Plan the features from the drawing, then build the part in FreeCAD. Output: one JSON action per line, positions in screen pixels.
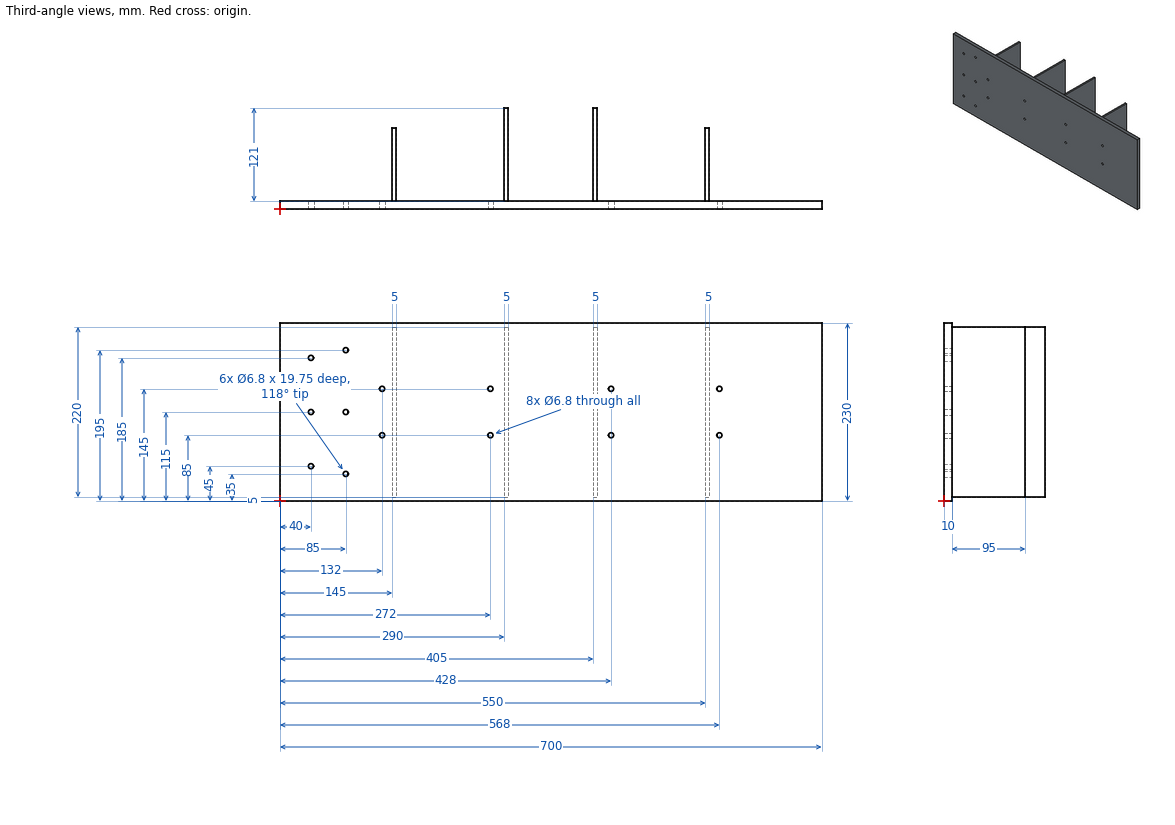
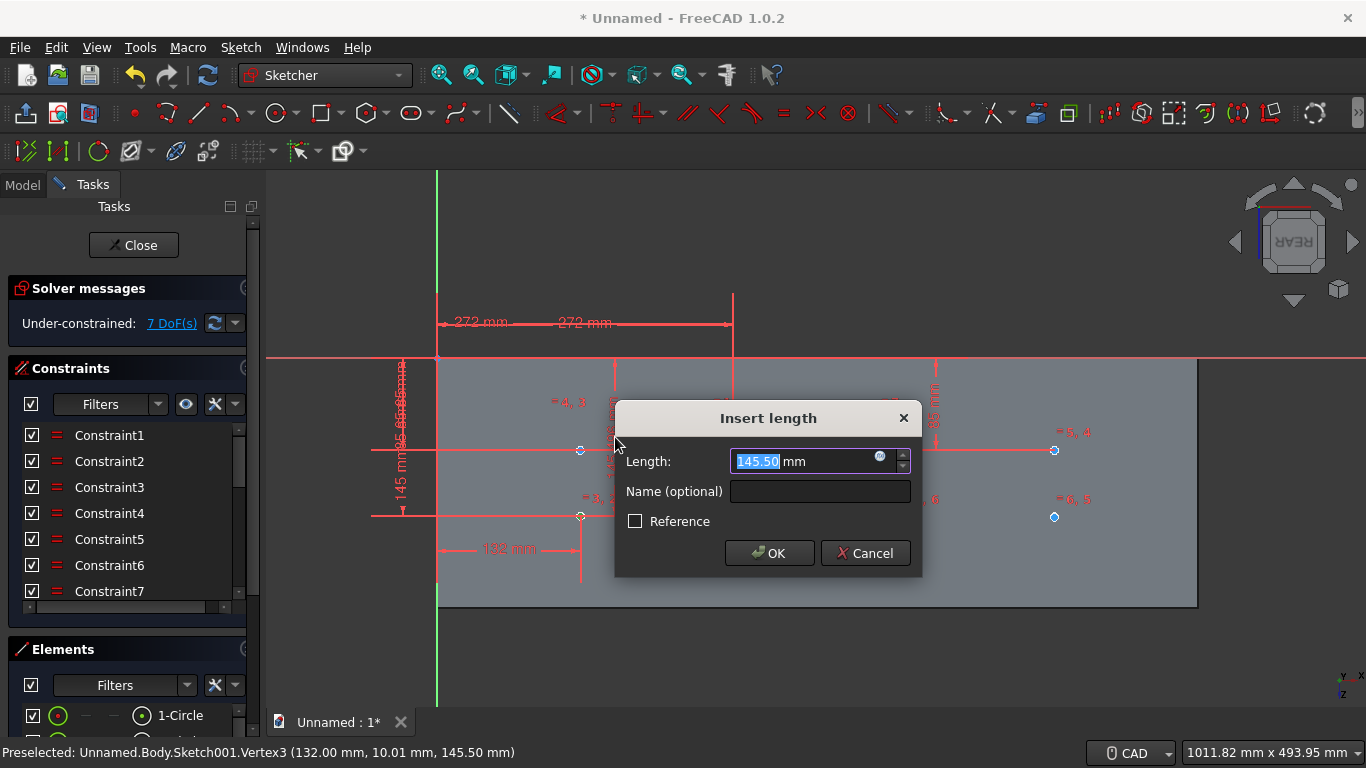
{"action": "type", "text": "145"}
{"action": "key", "text": "Return"}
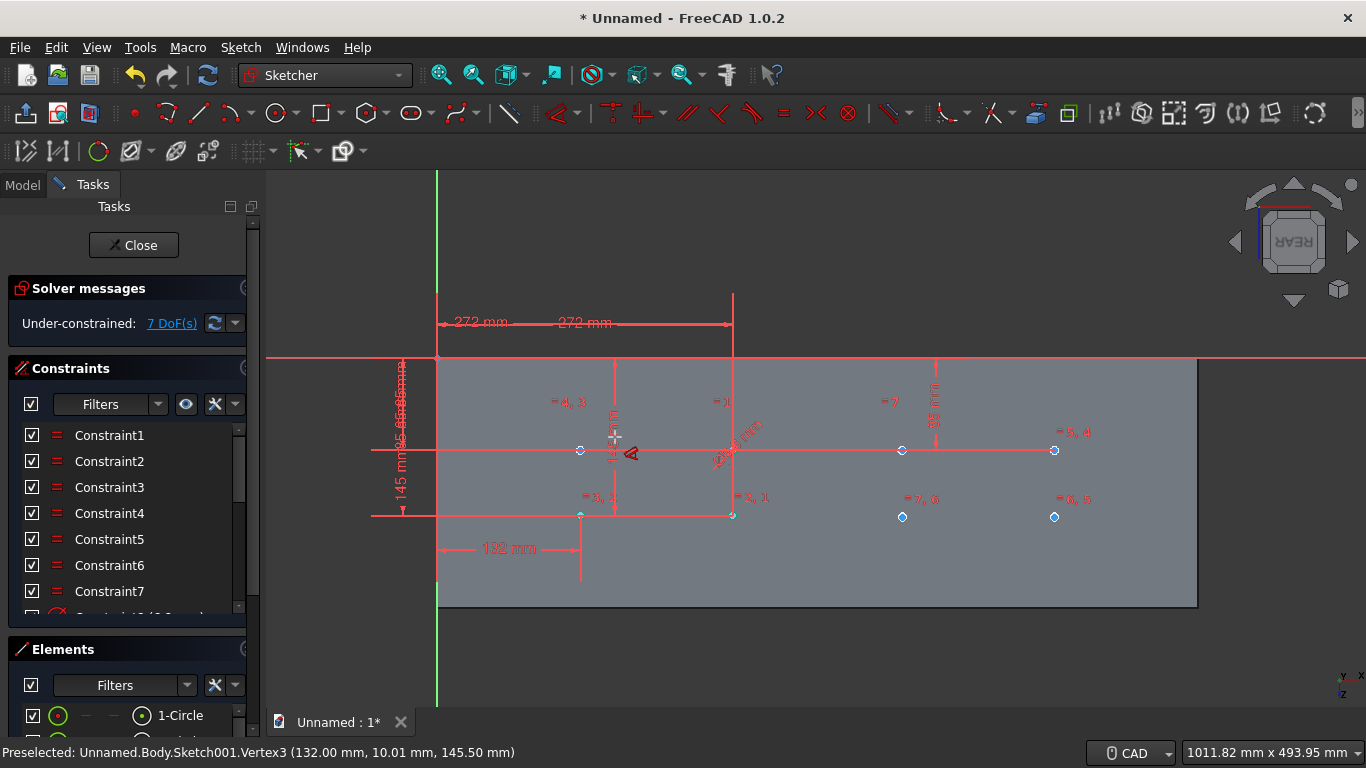
{"action": "left_click", "coordinate": [580, 450]}
{"action": "left_click", "coordinate": [509, 484]}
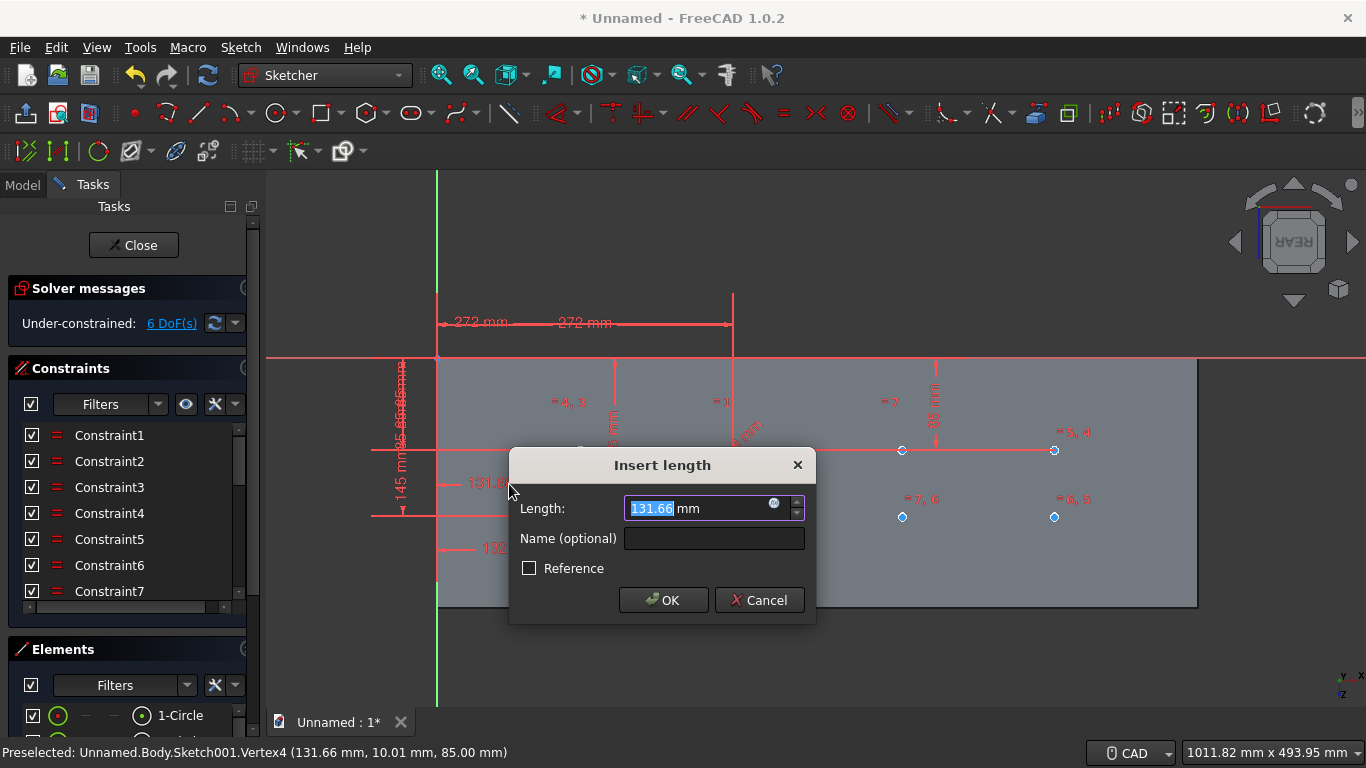
{"action": "type", "text": "132"}
{"action": "key", "text": "Return"}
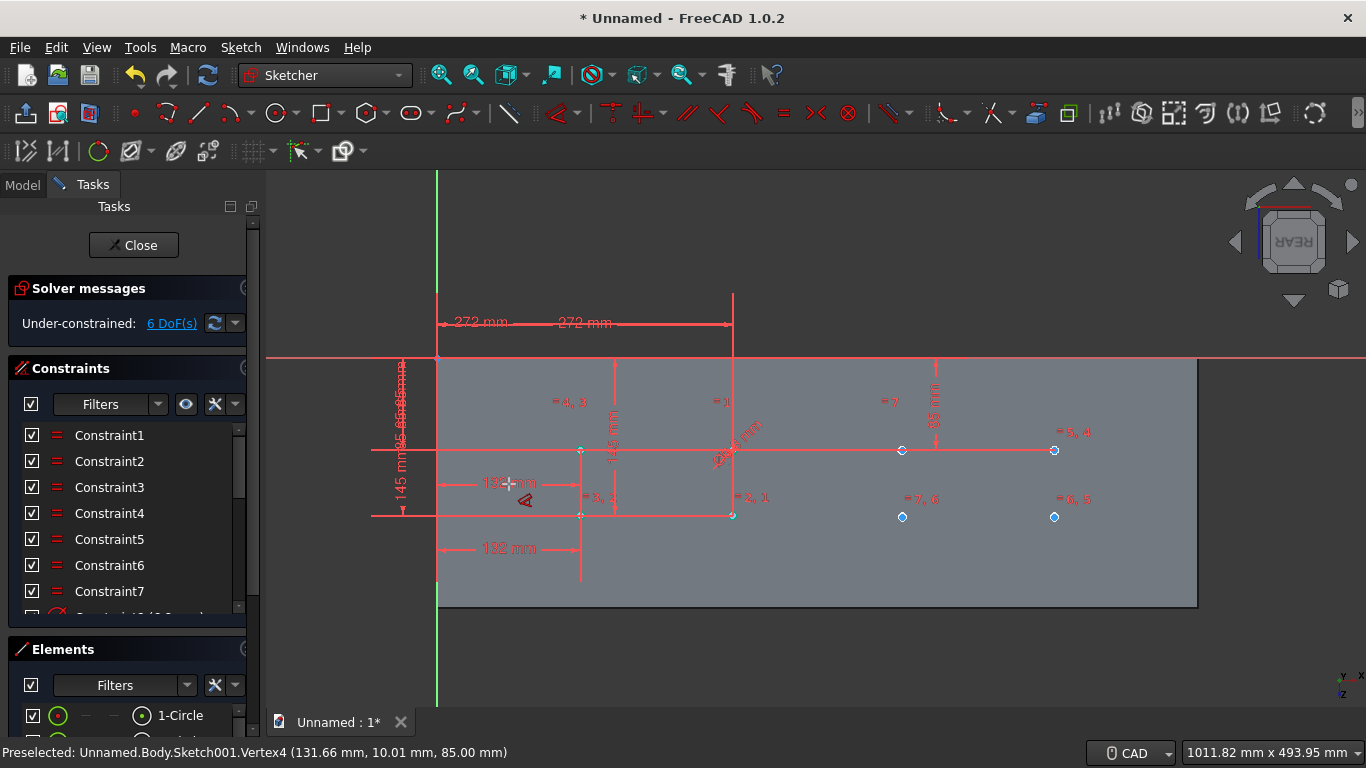
{"action": "left_click", "coordinate": [1054, 450]}
{"action": "left_click", "coordinate": [746, 324]}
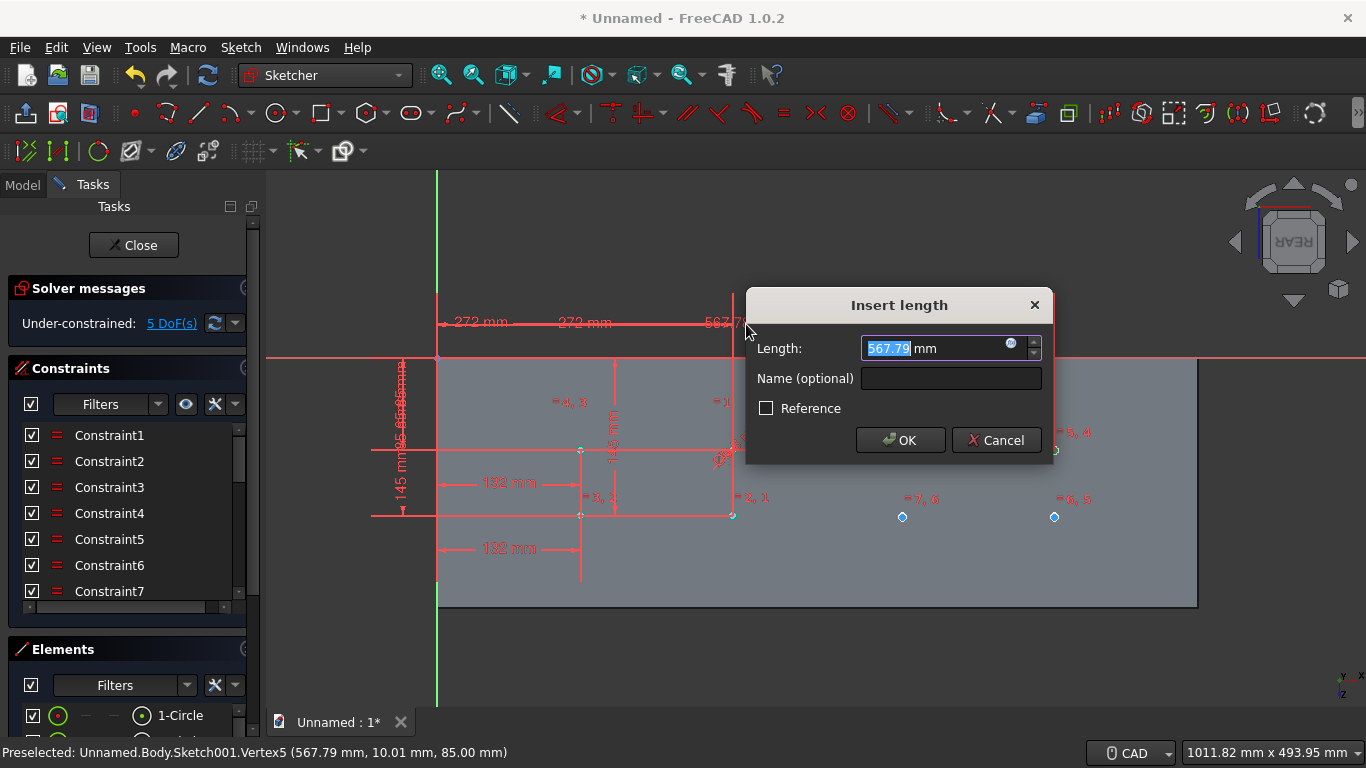
{"action": "type", "text": "568"}
{"action": "key", "text": "Return"}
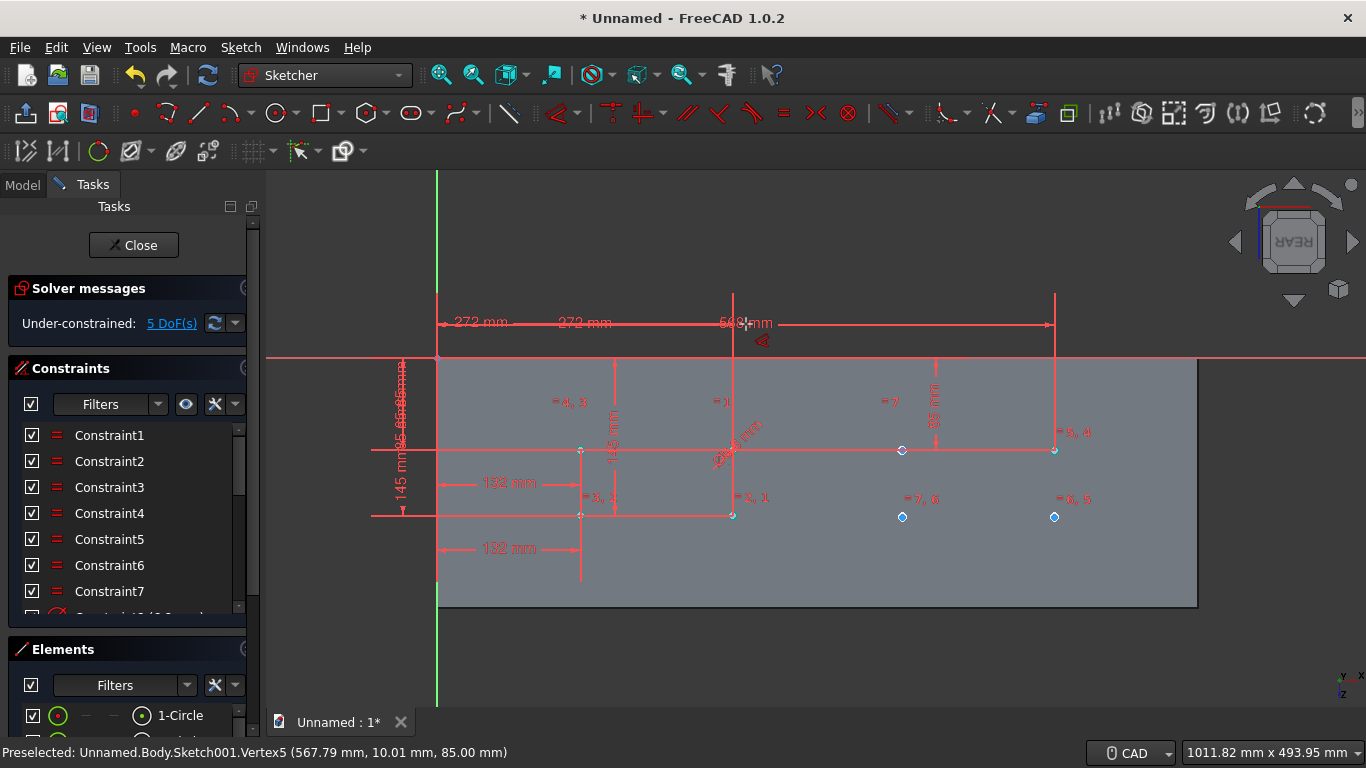
{"action": "left_click", "coordinate": [1054, 517]}
{"action": "left_click", "coordinate": [888, 324]}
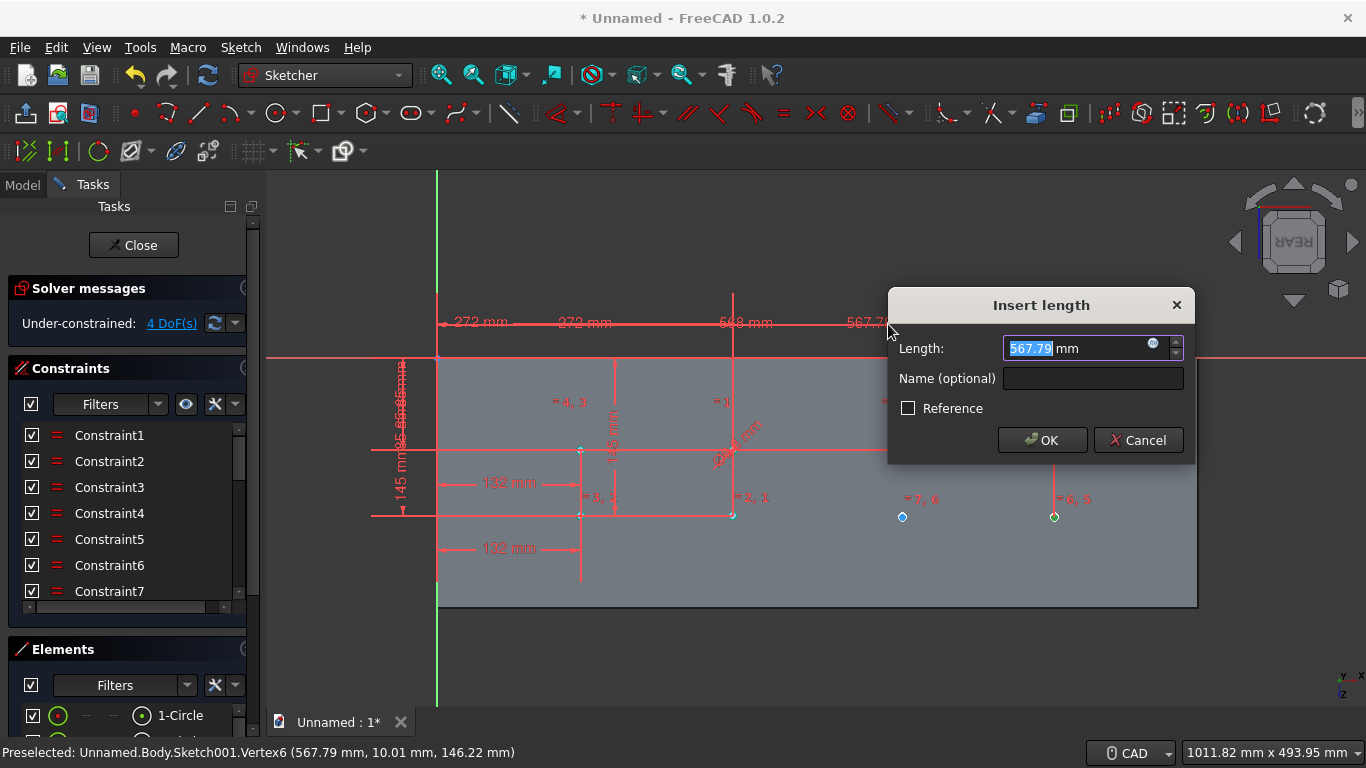
{"action": "type", "text": "568"}
{"action": "key", "text": "Return"}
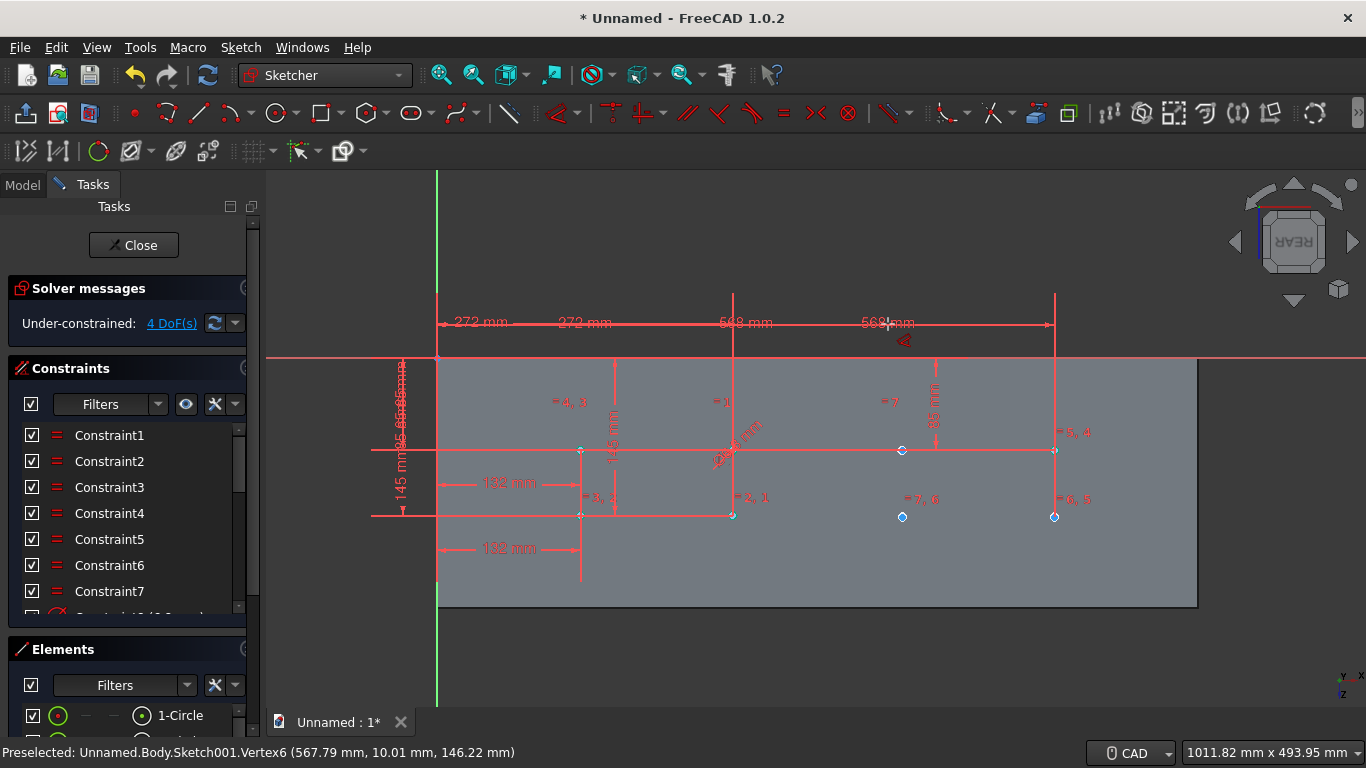
{"action": "left_click", "coordinate": [1055, 517]}
{"action": "left_click", "coordinate": [1089, 438]}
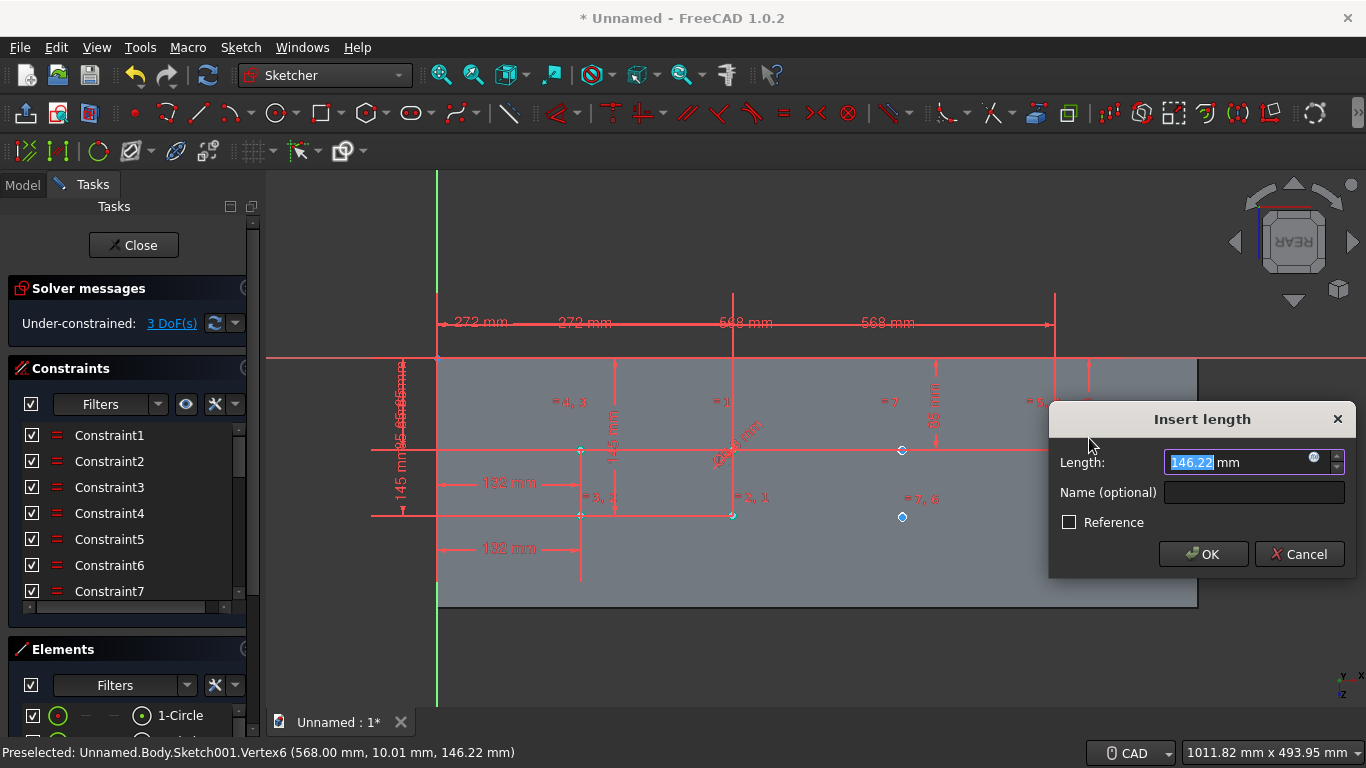
{"action": "type", "text": "145"}
{"action": "key", "text": "Return"}